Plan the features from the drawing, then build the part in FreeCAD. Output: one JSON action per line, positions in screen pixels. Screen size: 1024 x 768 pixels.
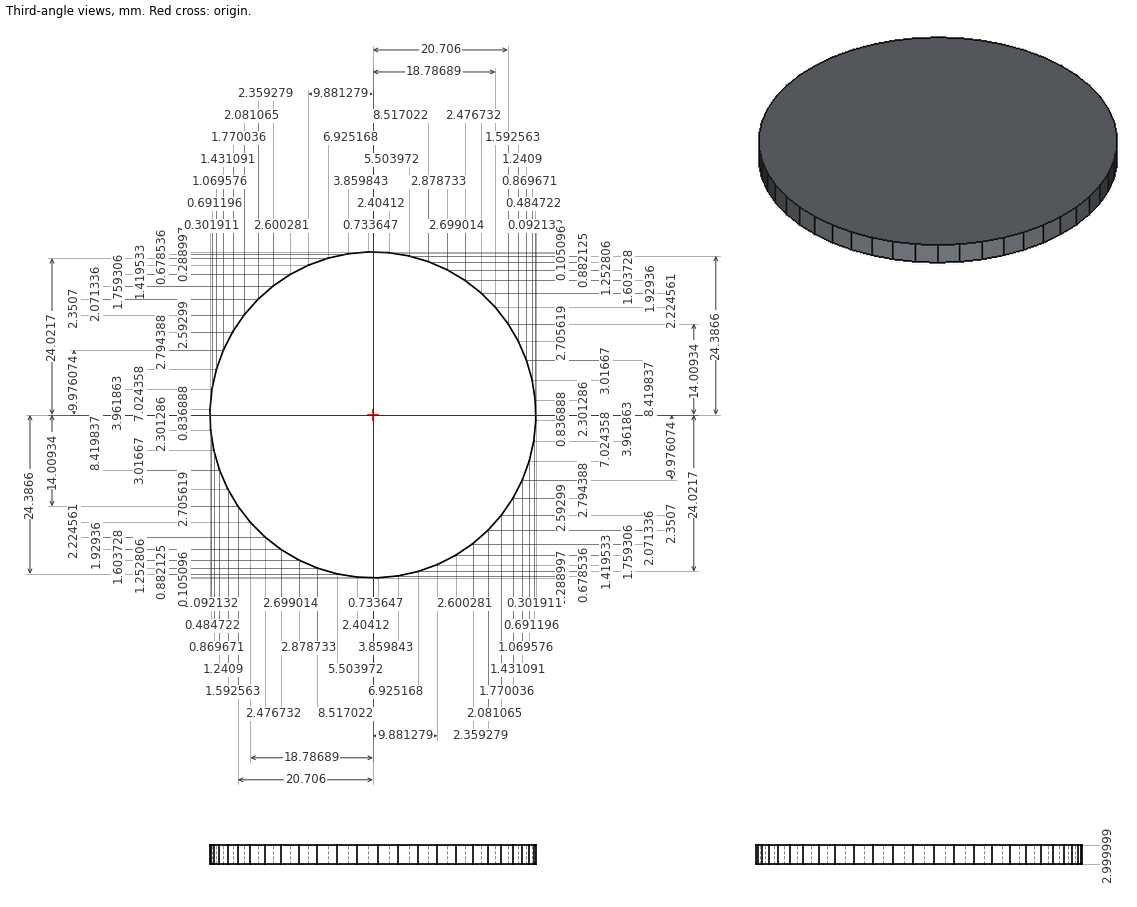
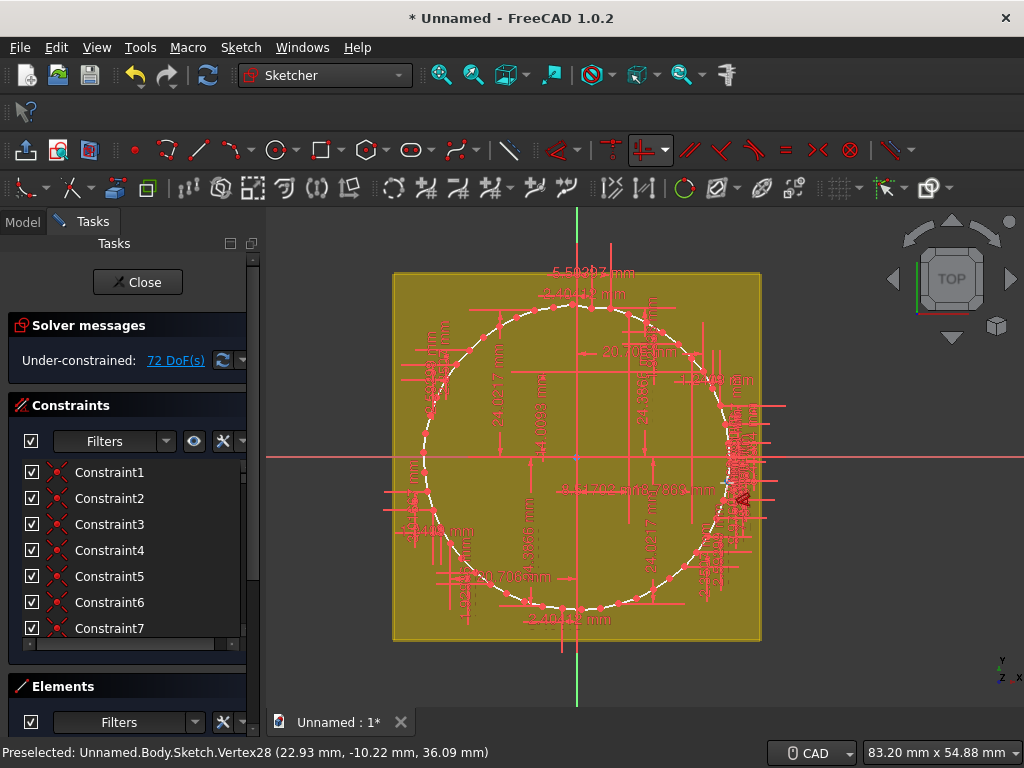
{"action": "left_click", "coordinate": [637, 599]}
{"action": "left_click", "coordinate": [621, 423]}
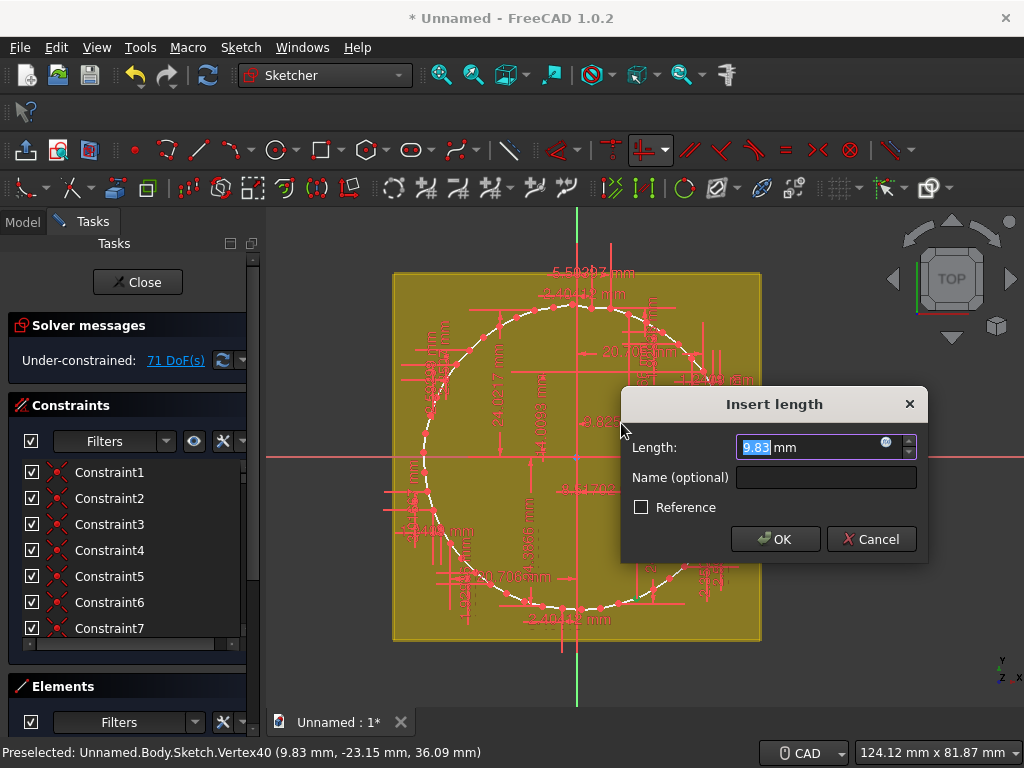
{"action": "type", "text": "9.881279"}
{"action": "key", "text": "Return"}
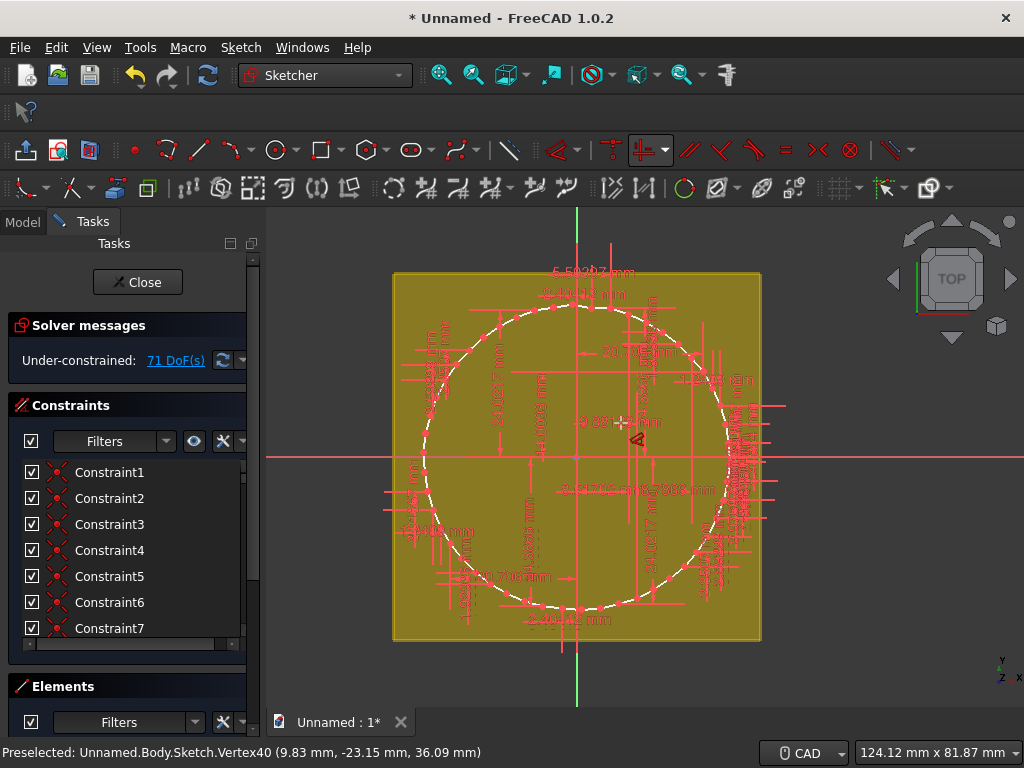
{"action": "left_click", "coordinate": [619, 604]}
{"action": "left_click", "coordinate": [598, 662]}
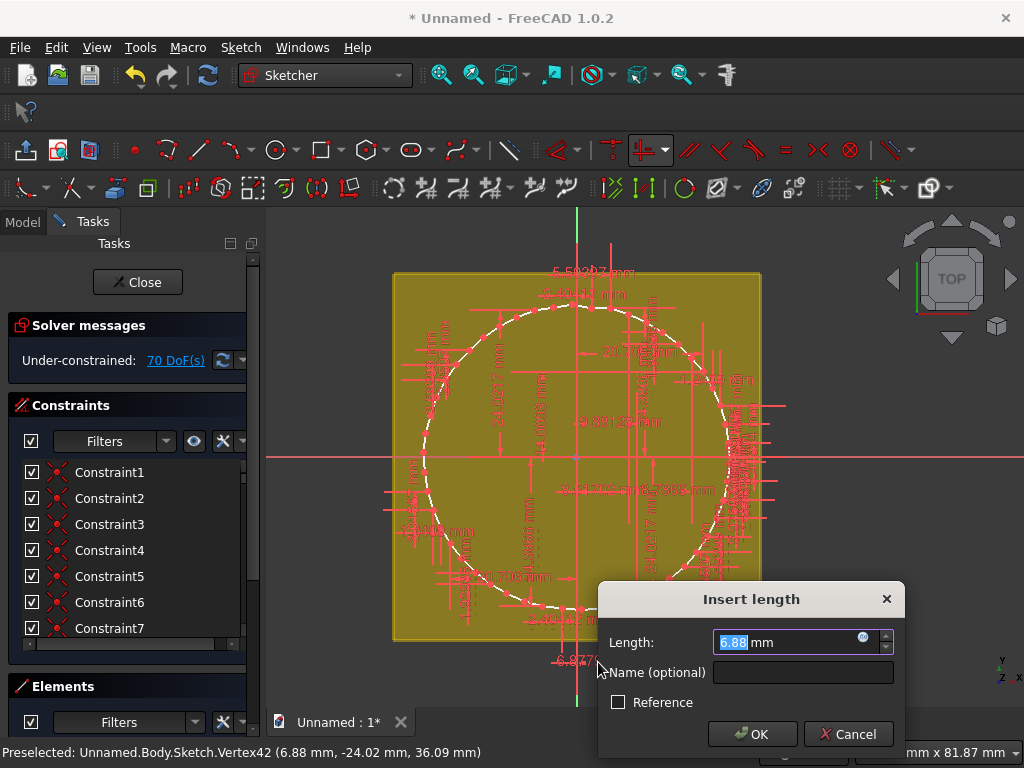
{"action": "type", "text": "6.925168"}
{"action": "key", "text": "Return"}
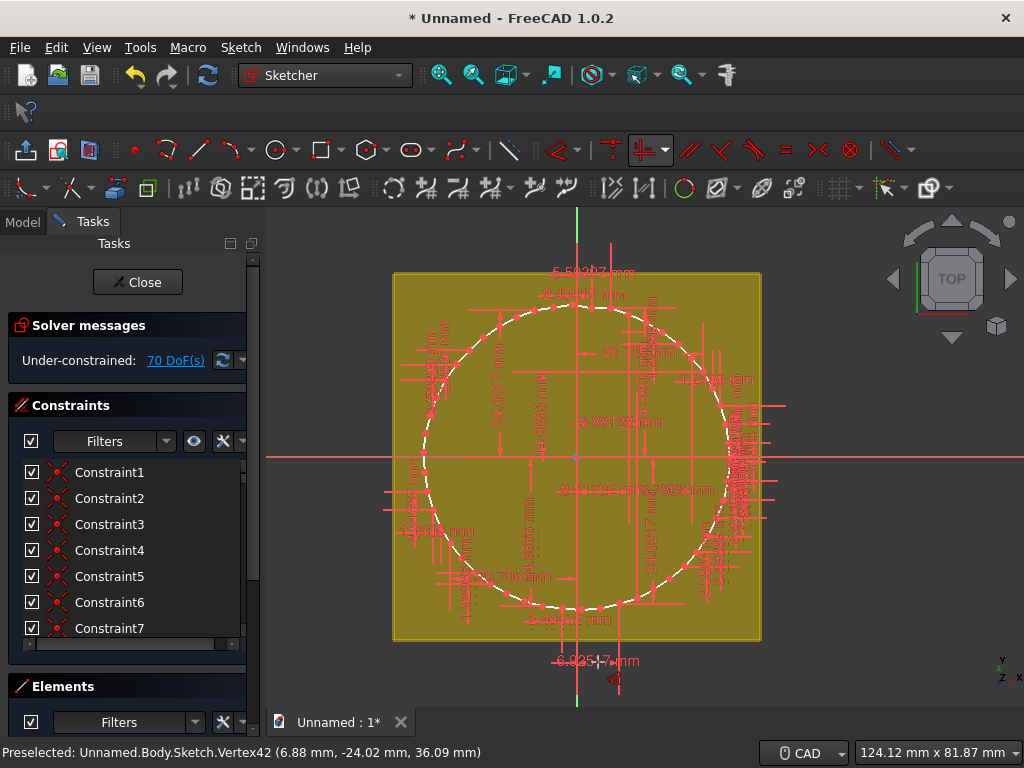
{"action": "scroll", "coordinate": [601, 609], "scroll_direction": "up", "scroll_amount": 3}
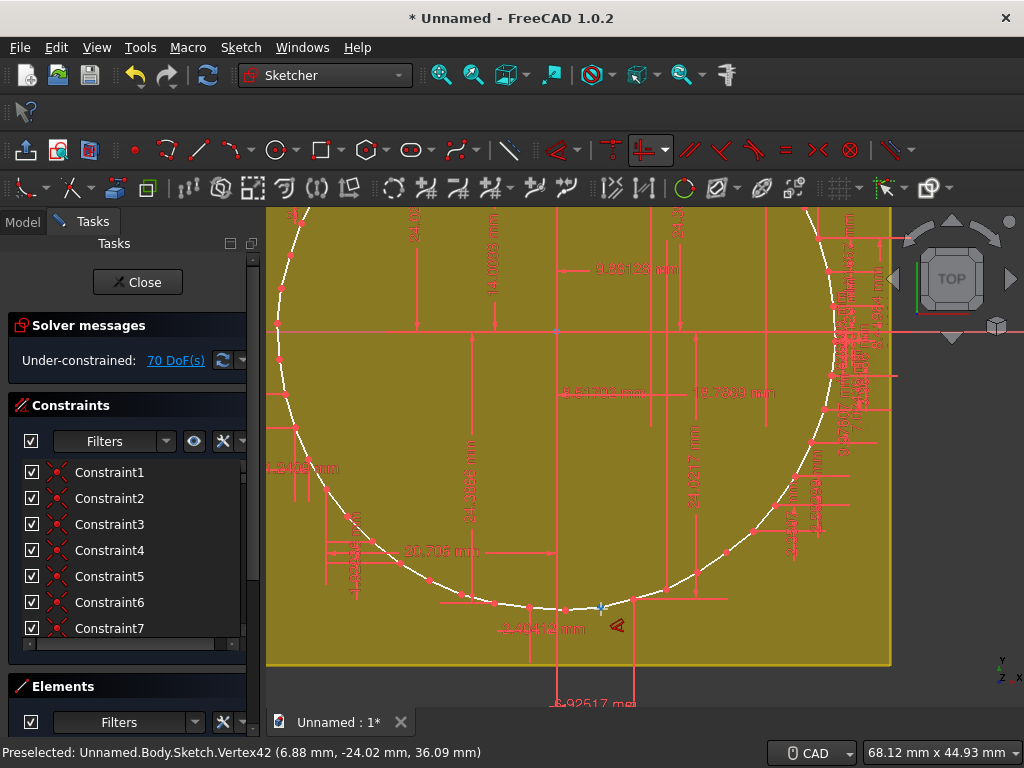
{"action": "left_click", "coordinate": [600, 608]}
{"action": "left_click", "coordinate": [579, 298]}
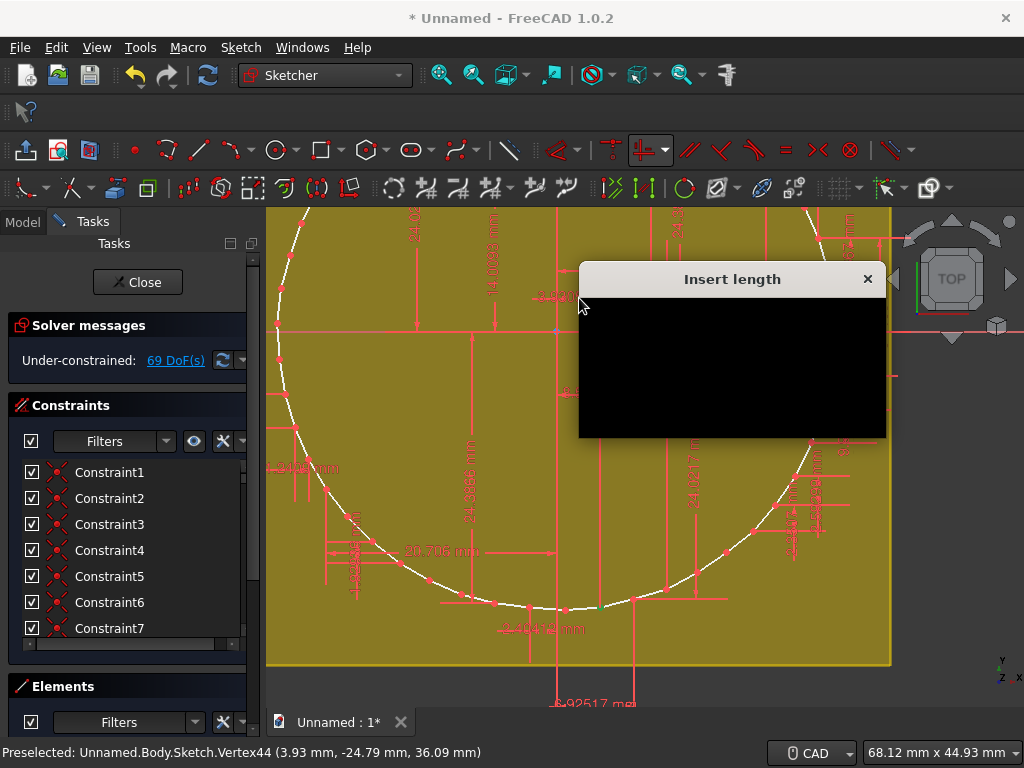
{"action": "type", "text": "3.859843"}
{"action": "key", "text": "Return"}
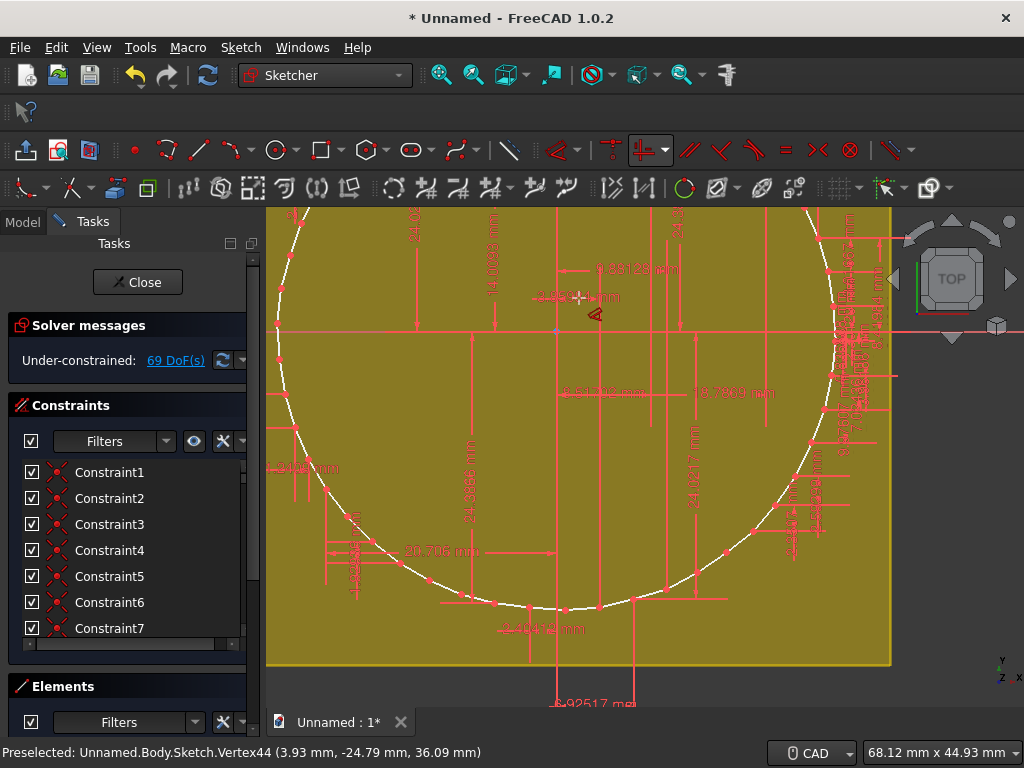
{"action": "scroll", "coordinate": [565, 610], "scroll_direction": "up", "scroll_amount": 8}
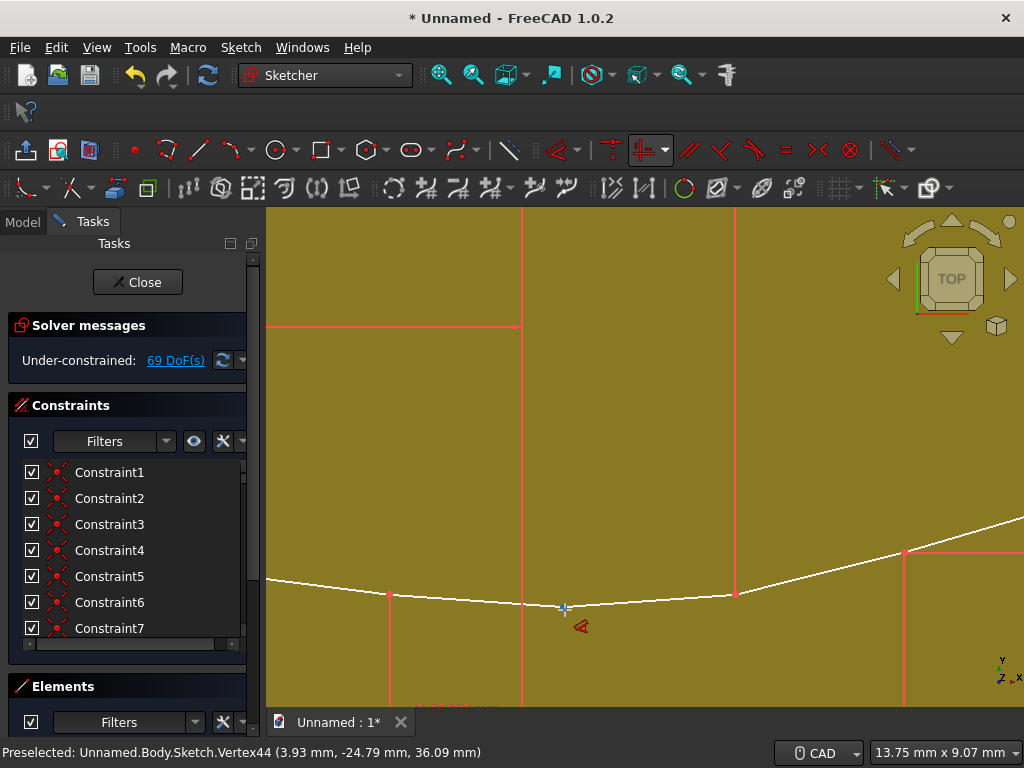
{"action": "left_click", "coordinate": [564, 607]}
{"action": "left_click", "coordinate": [543, 641]}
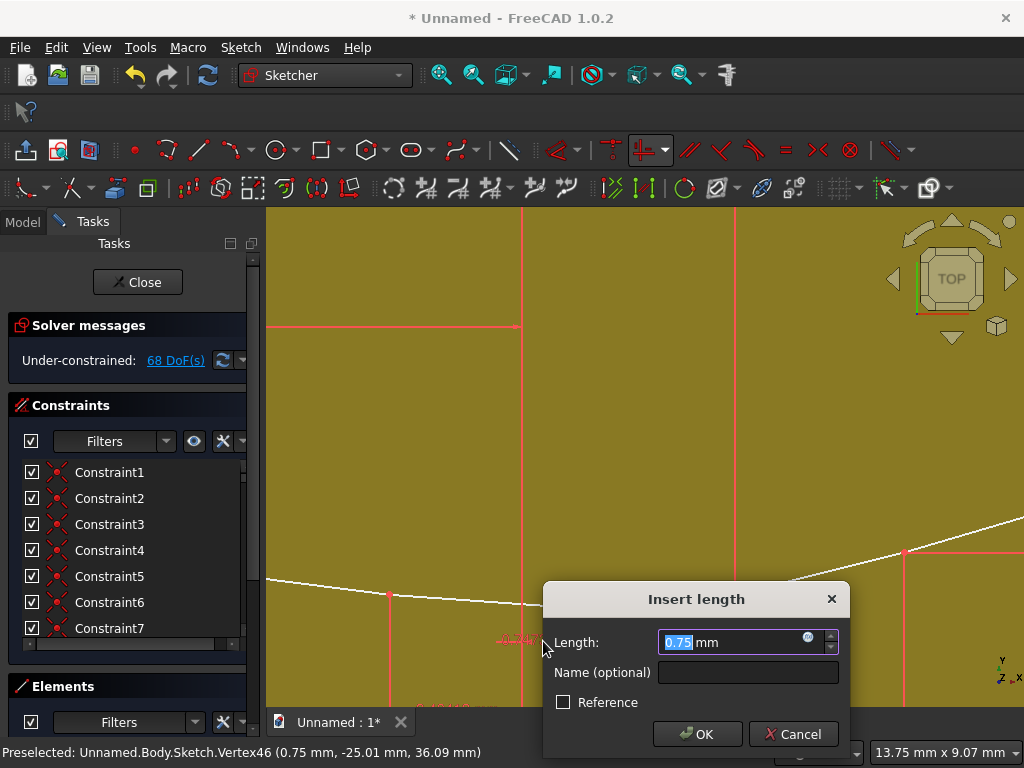
{"action": "type", "text": "0.733647"}
{"action": "key", "text": "Return"}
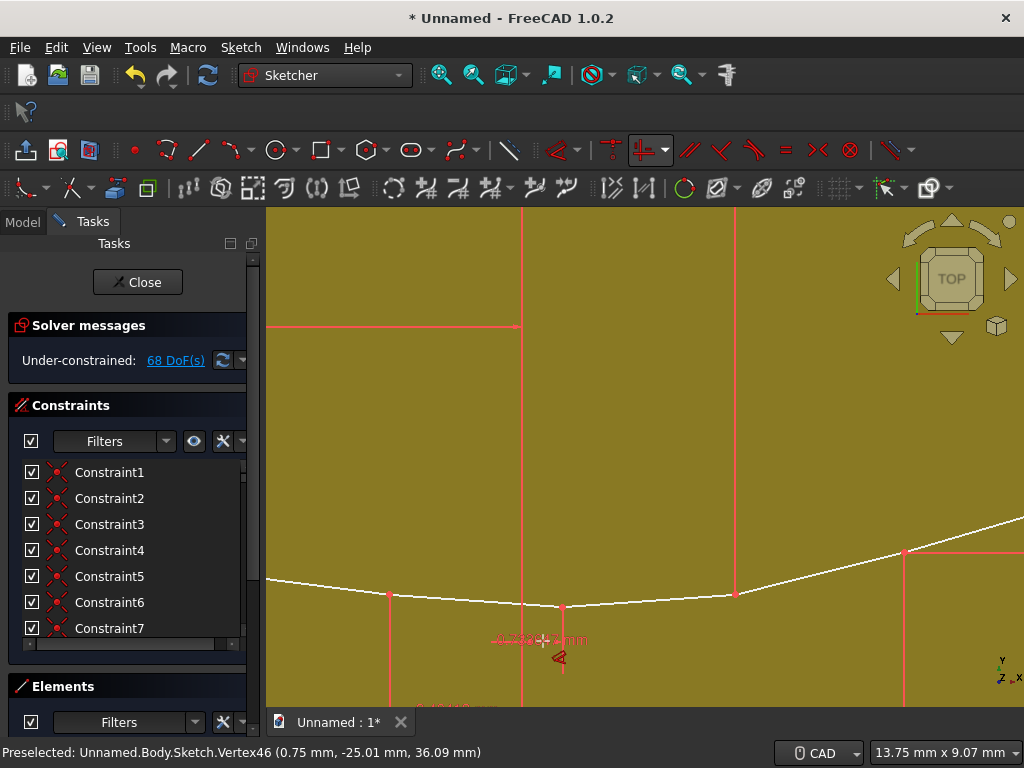
{"action": "scroll", "coordinate": [583, 610], "scroll_direction": "down", "scroll_amount": 11}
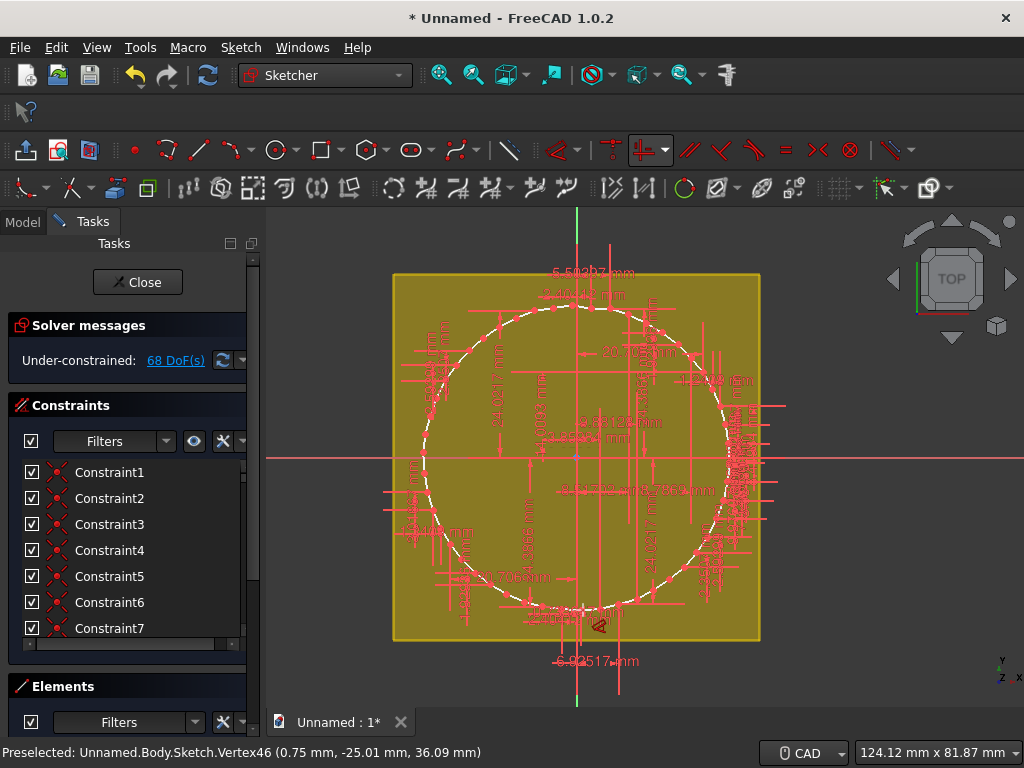
{"action": "left_click", "coordinate": [543, 607]}
{"action": "left_click", "coordinate": [560, 352]}